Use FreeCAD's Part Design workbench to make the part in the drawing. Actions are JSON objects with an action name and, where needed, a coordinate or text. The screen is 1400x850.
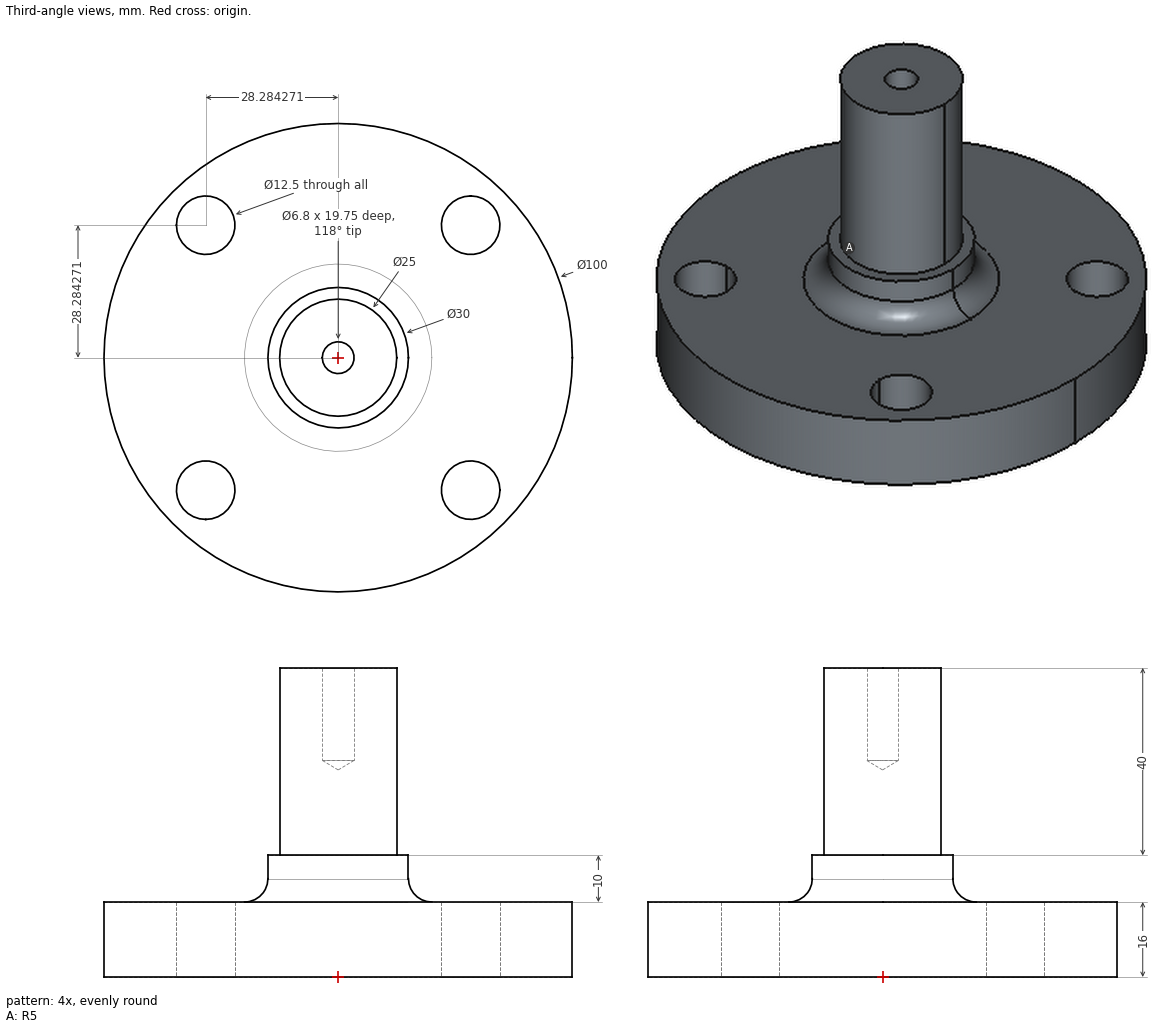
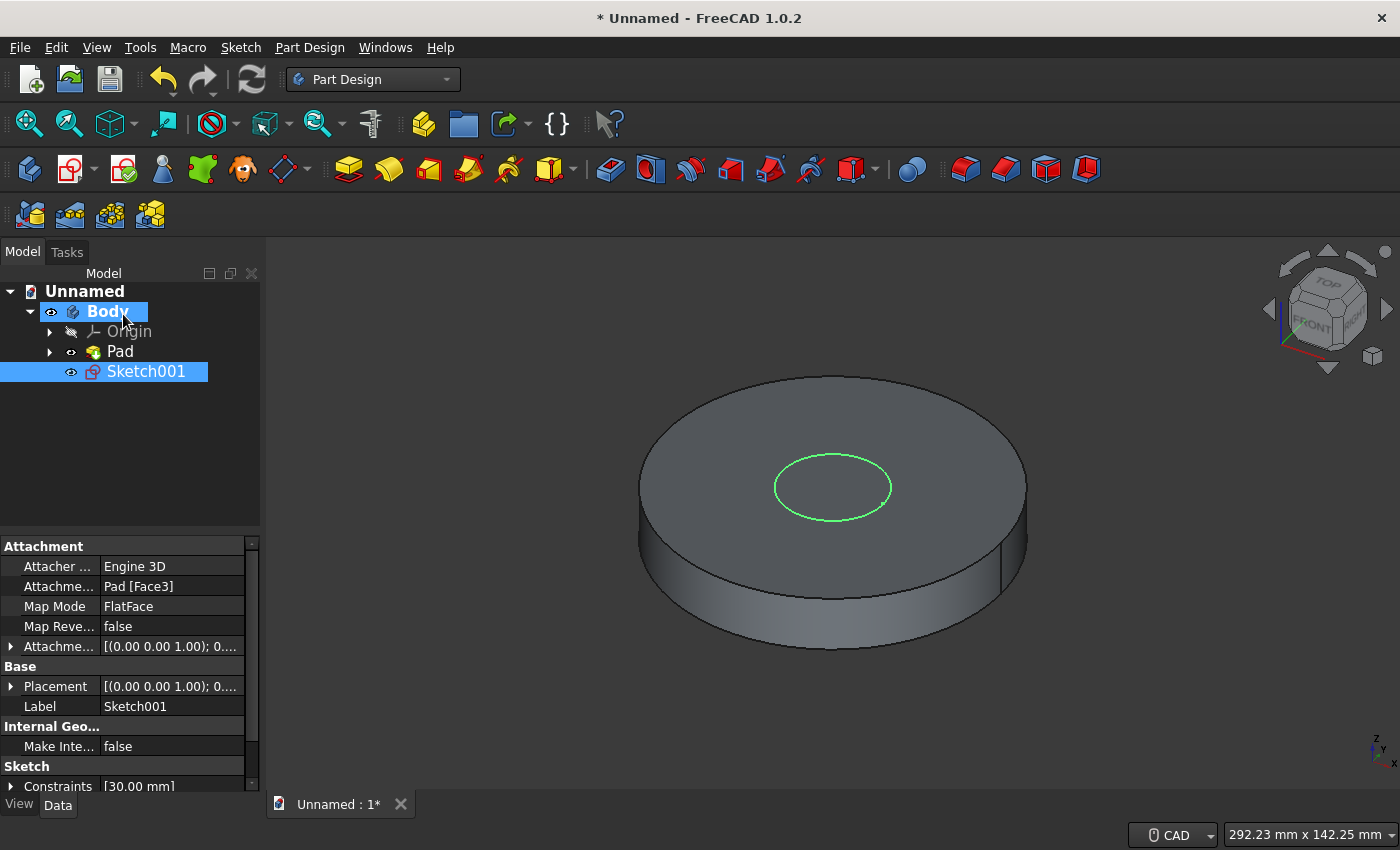
{"action": "left_click", "coordinate": [350, 170]}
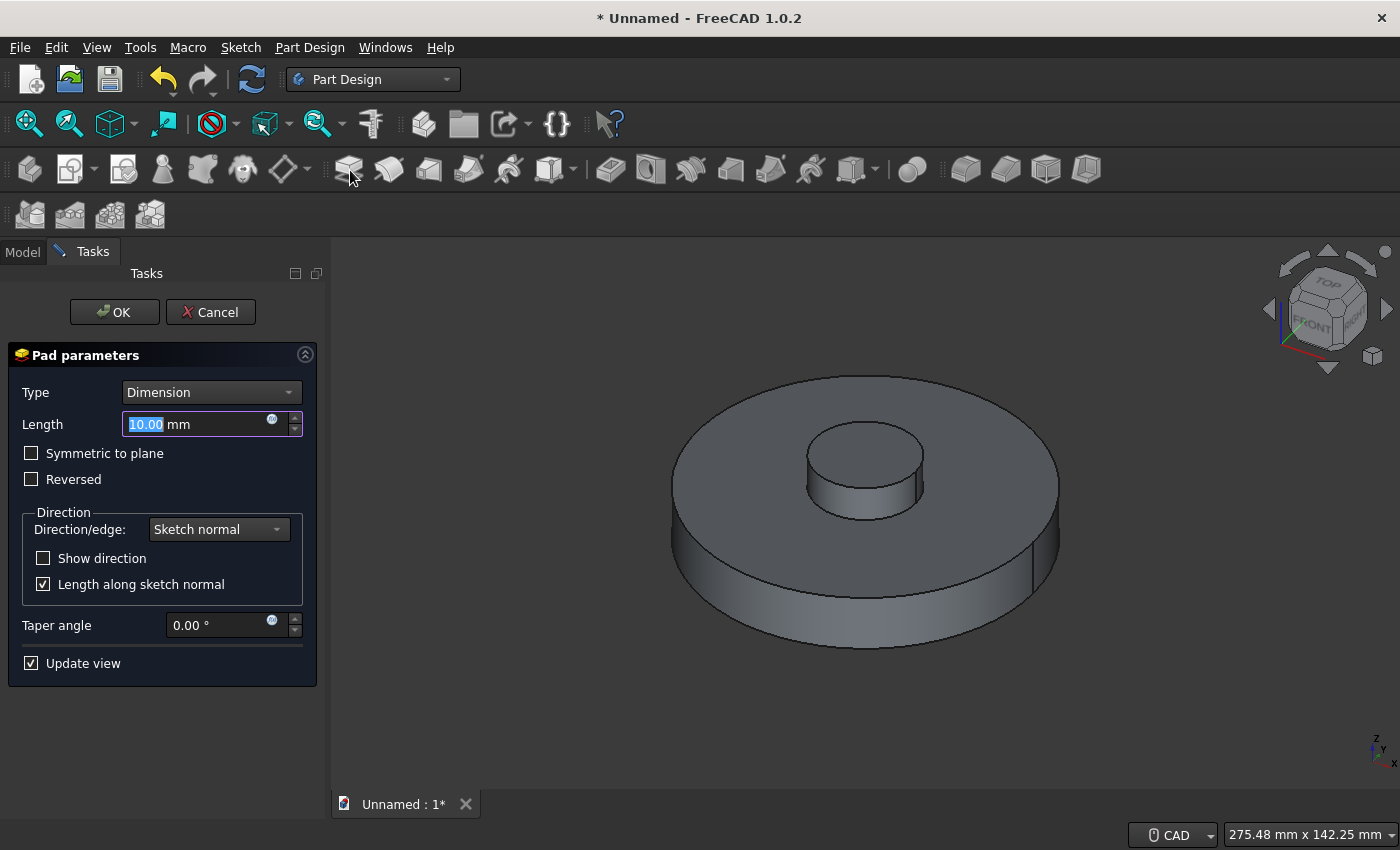
{"action": "type", "text": "10"}
{"action": "key", "text": "Tab"}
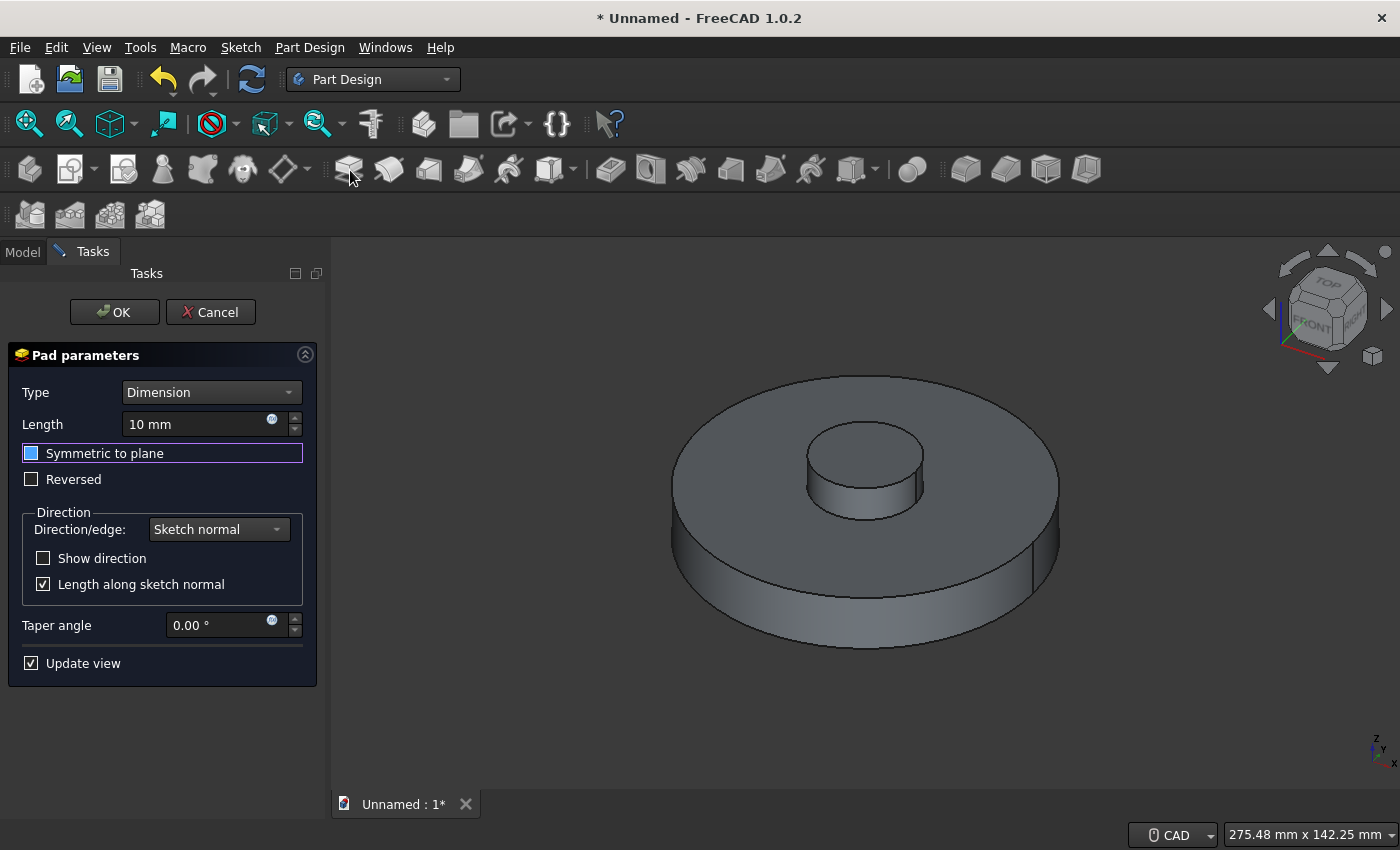
{"action": "left_click", "coordinate": [115, 312]}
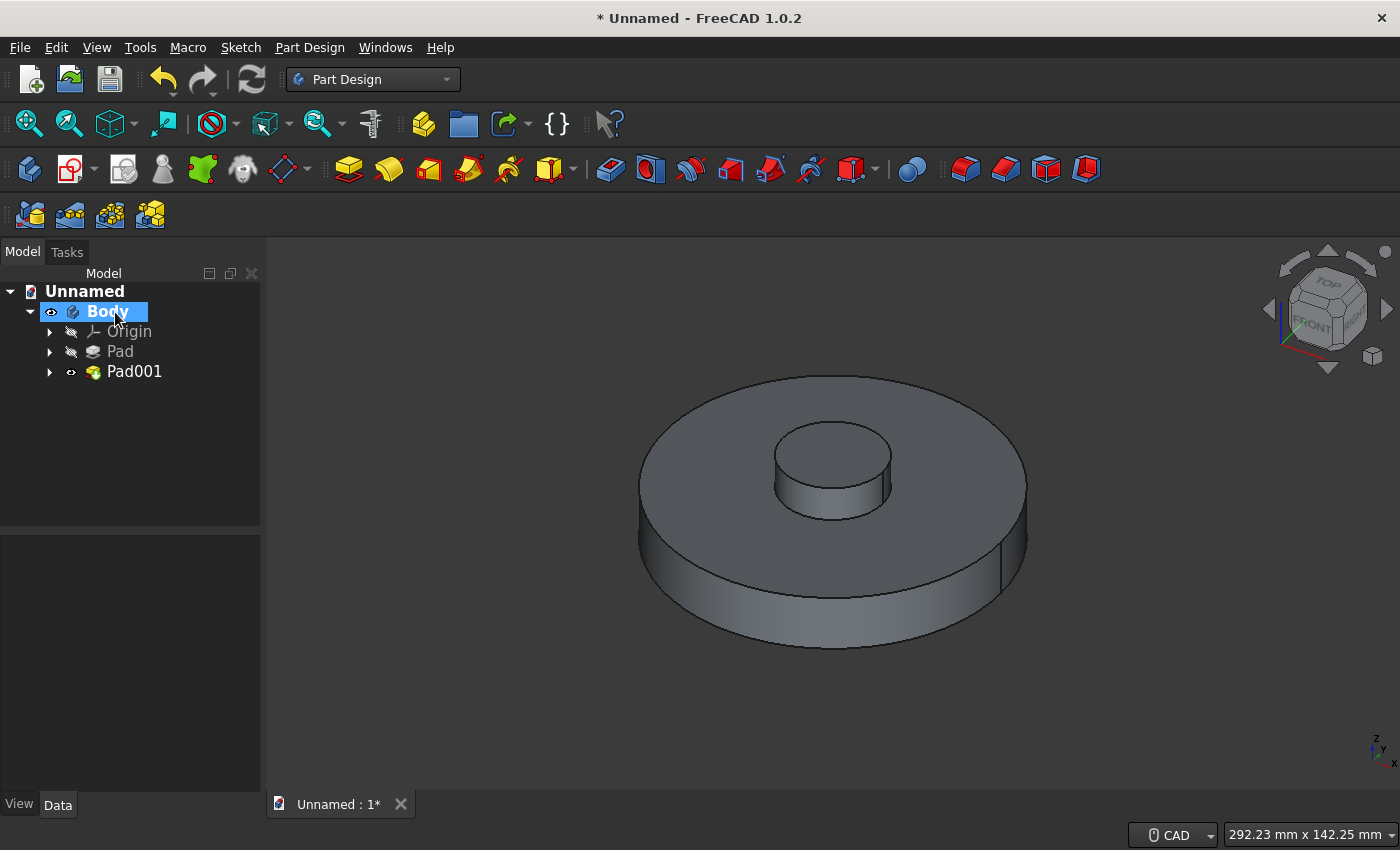
{"action": "left_click", "coordinate": [833, 454]}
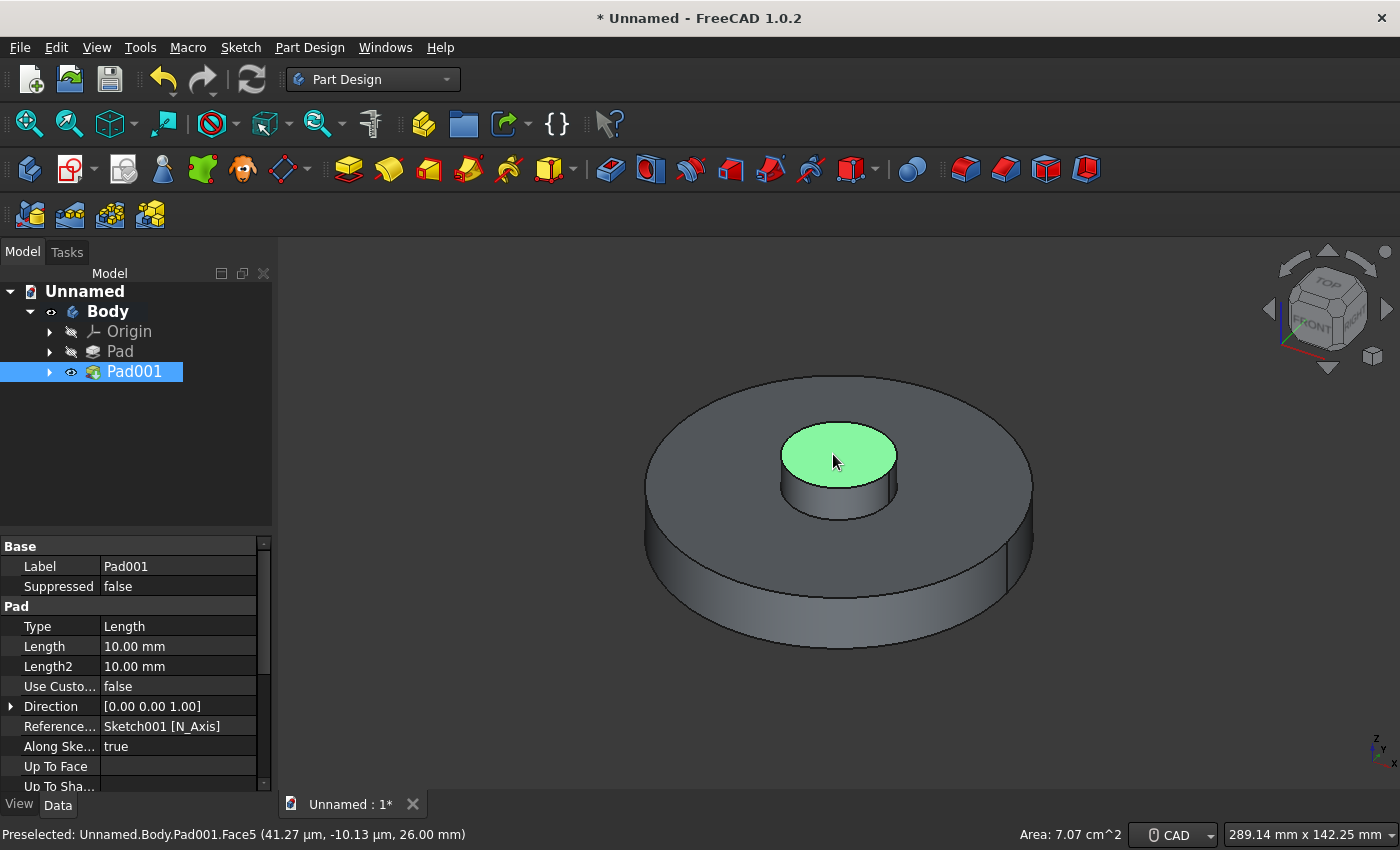
{"action": "left_click", "coordinate": [70, 170]}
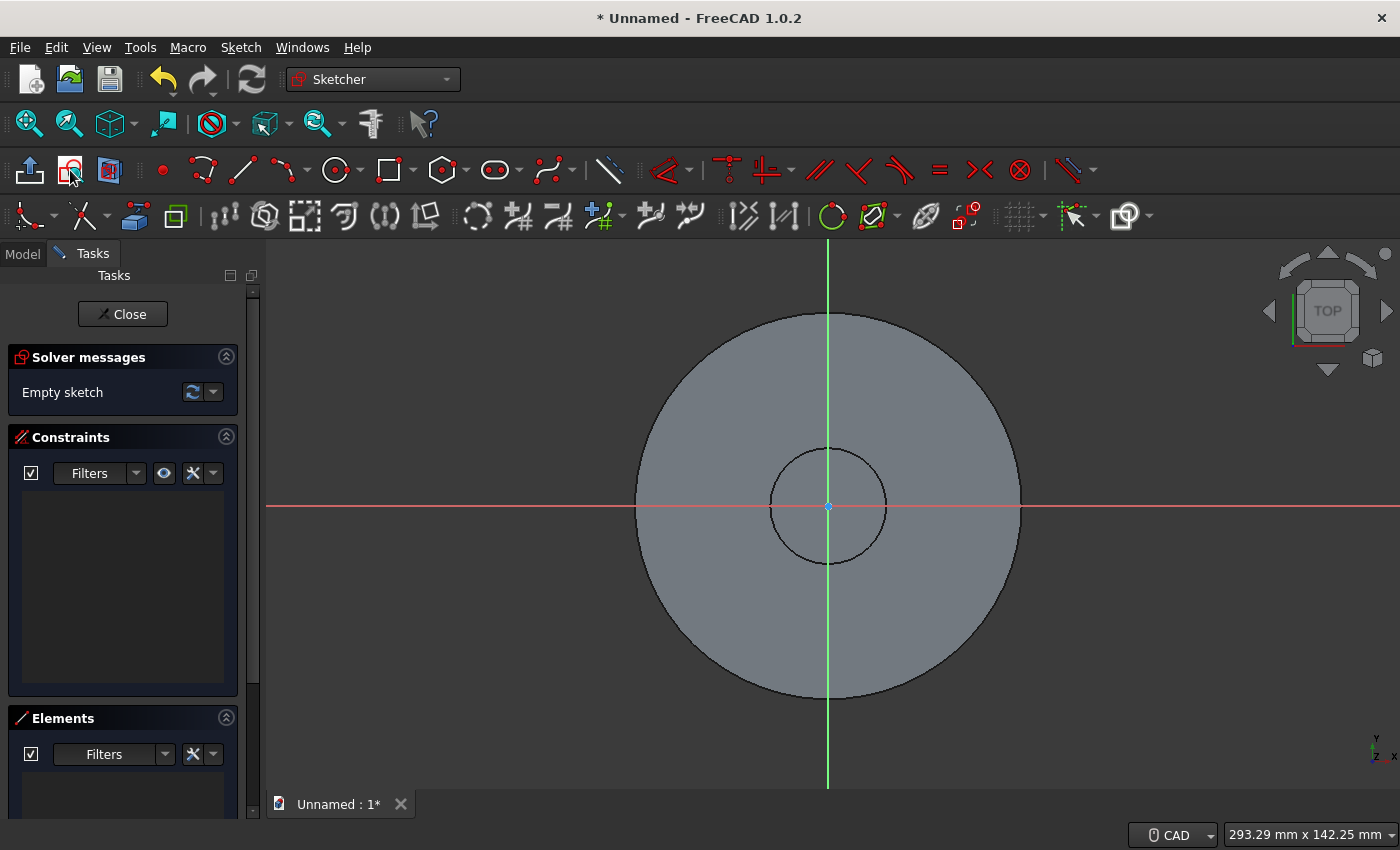
{"action": "scroll", "coordinate": [856, 503], "scroll_direction": "up", "scroll_amount": 6}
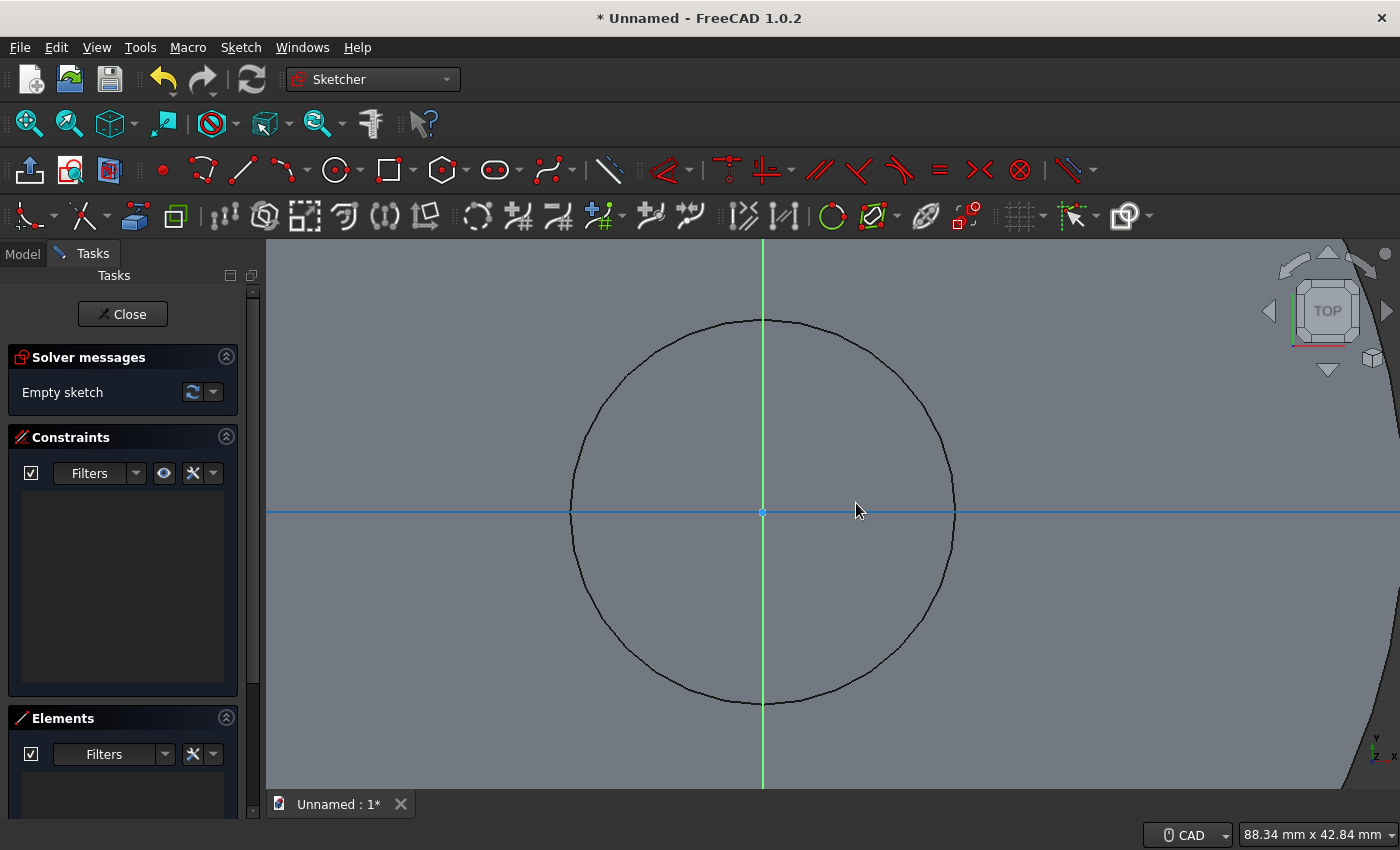
{"action": "key", "text": "g c"}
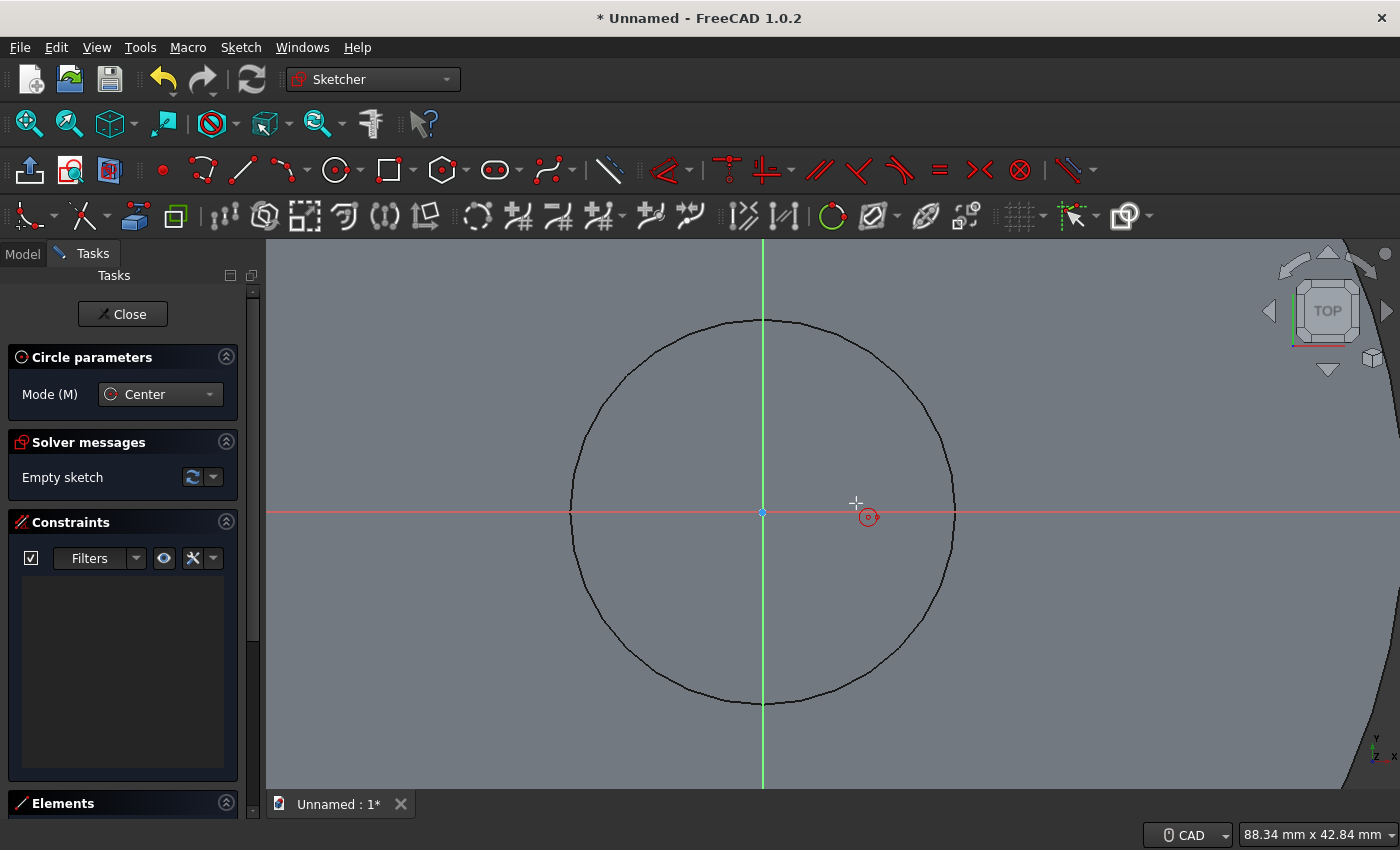
{"action": "left_click", "coordinate": [763, 512]}
{"action": "left_click", "coordinate": [876, 399]}
{"action": "key", "text": "Escape"}